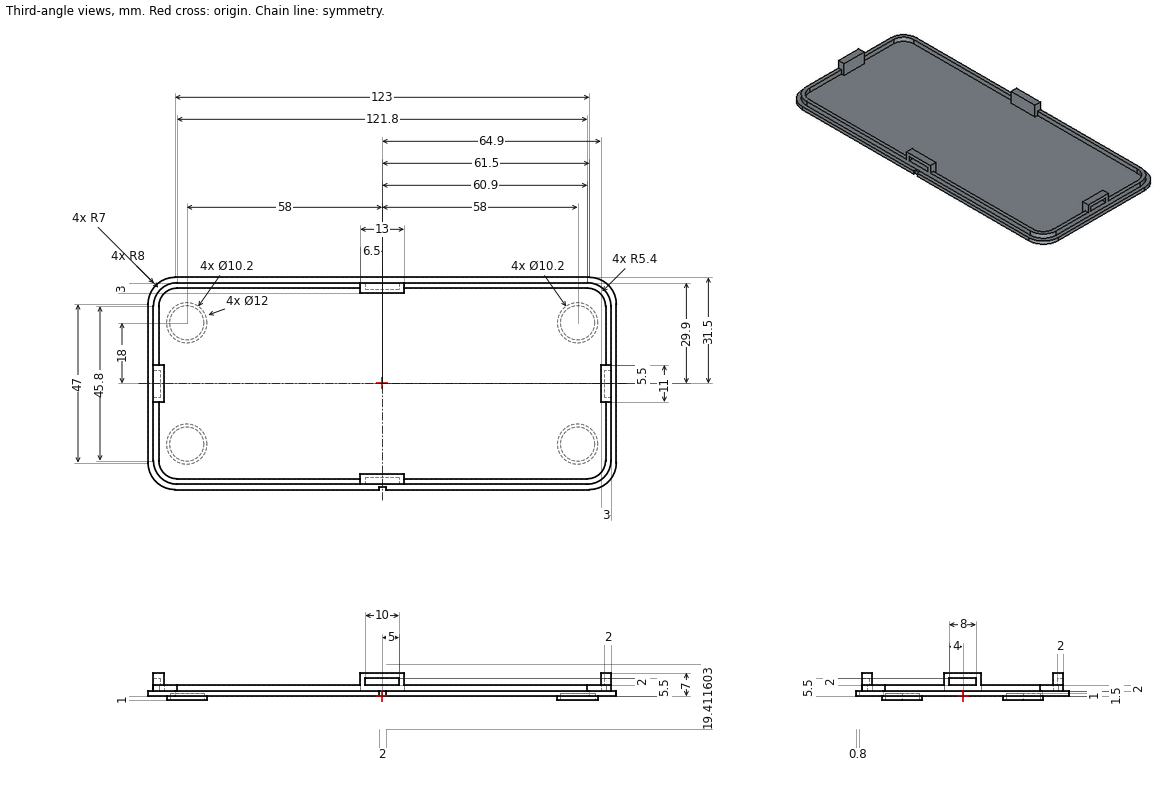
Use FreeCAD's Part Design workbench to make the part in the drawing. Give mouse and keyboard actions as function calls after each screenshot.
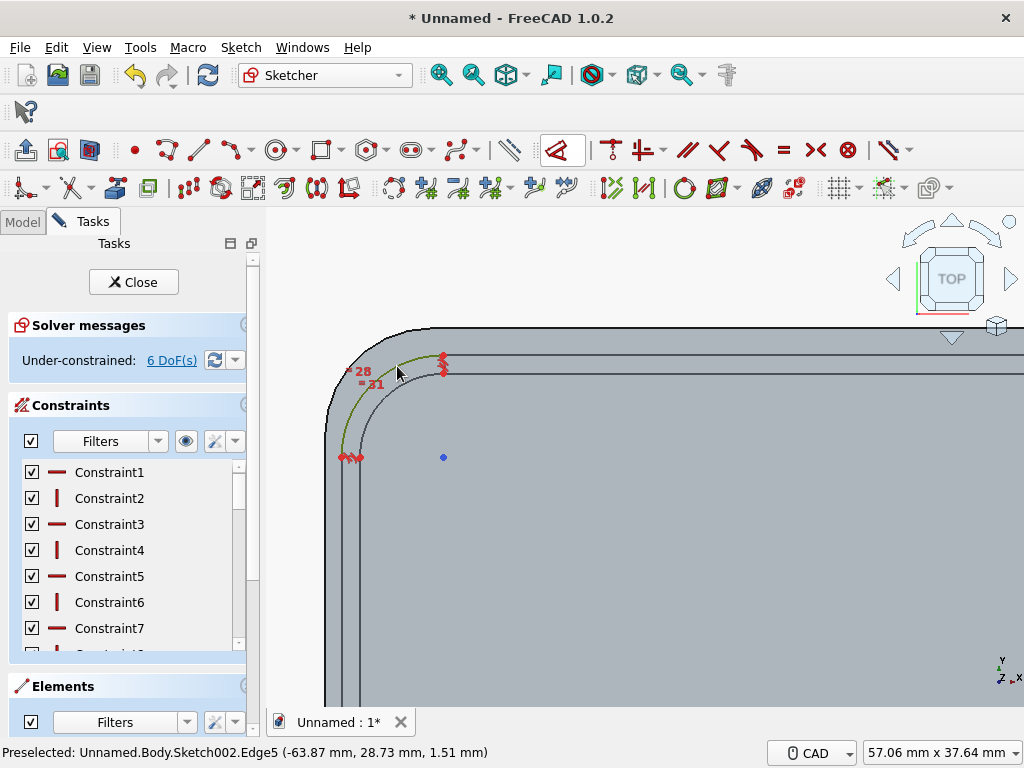
key(k)
key(r)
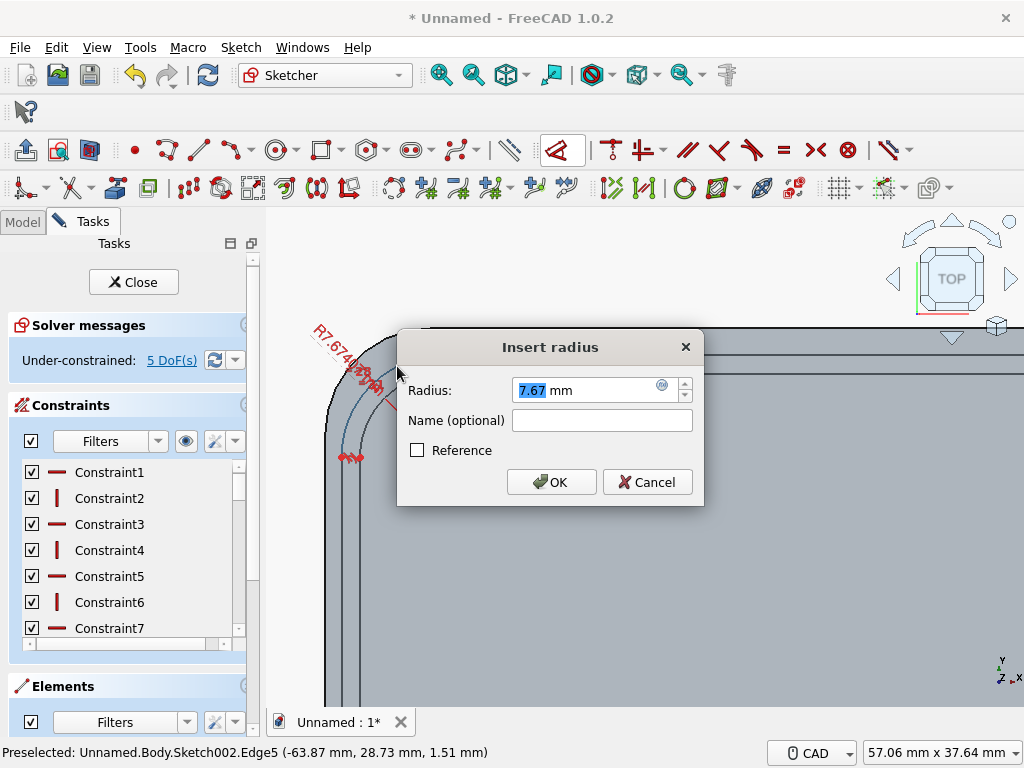
text(7)
key(Return)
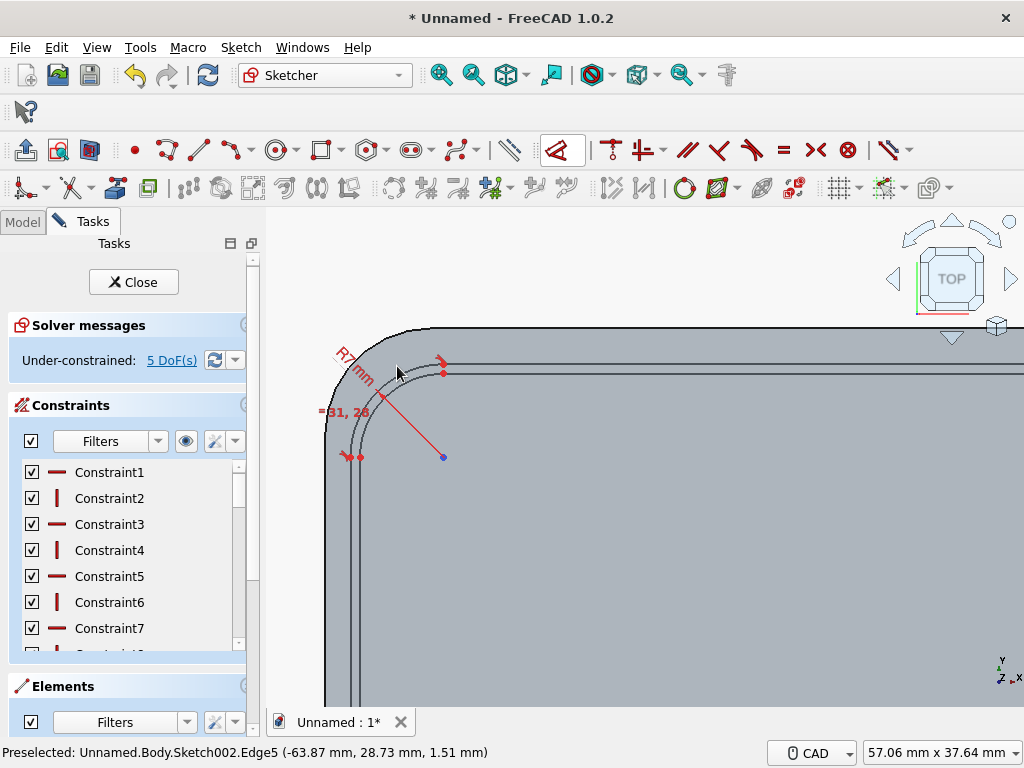
scroll(406, 384, down, 8)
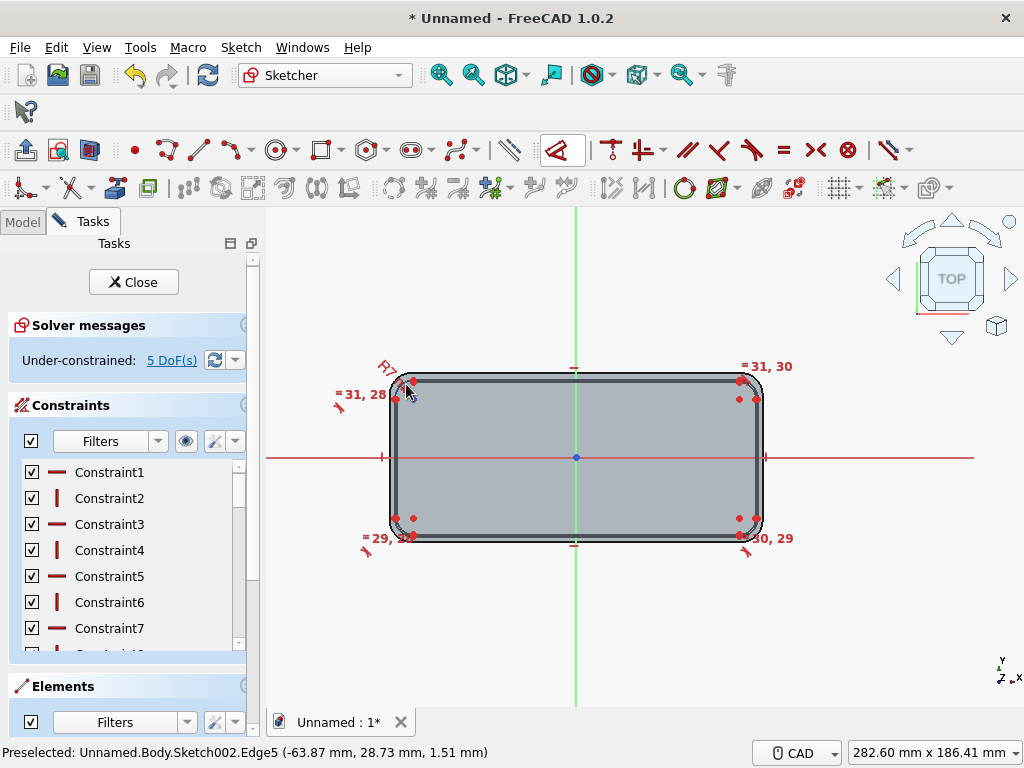
scroll(754, 391, up, 10)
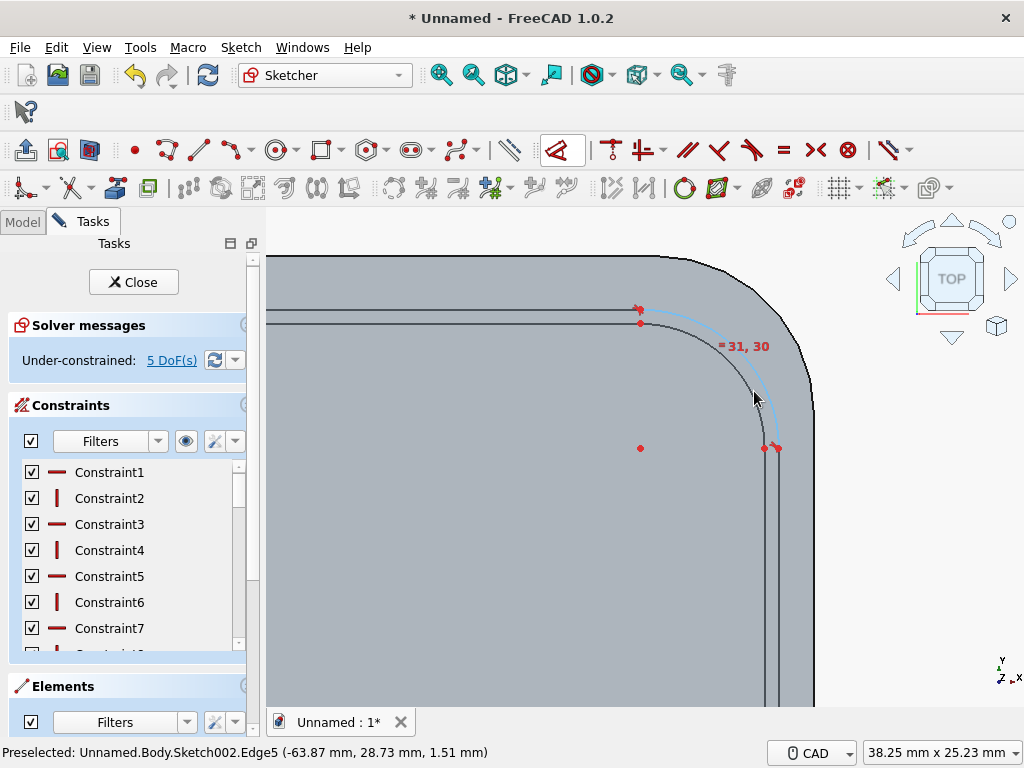
click(751, 392)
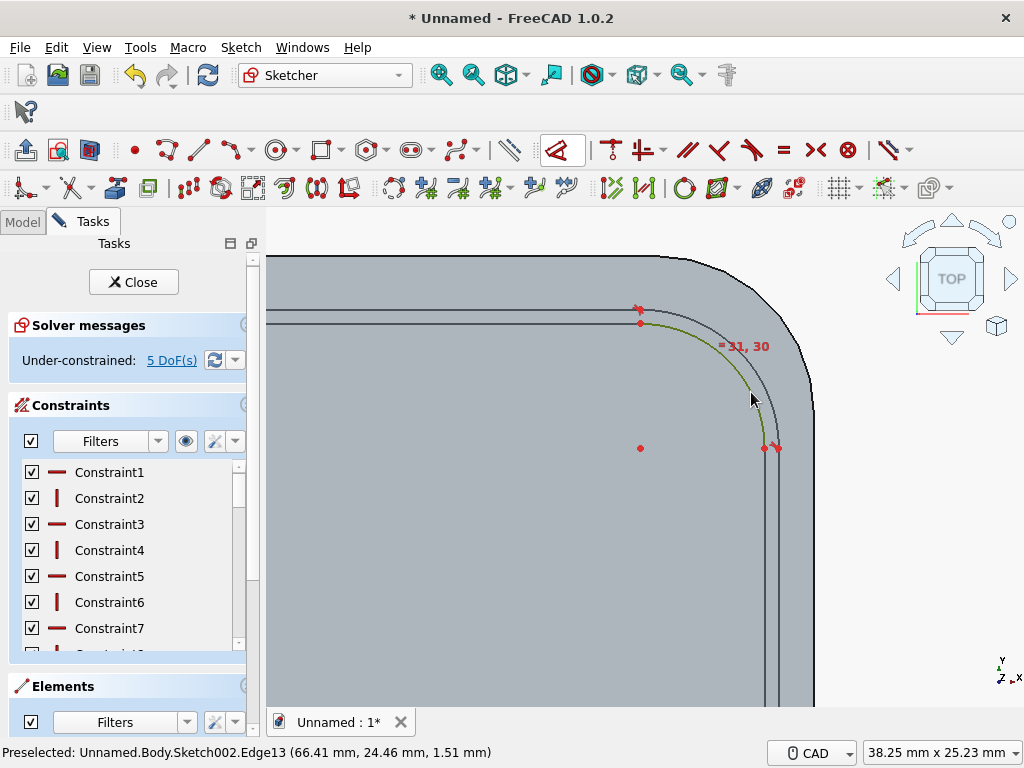
key(k)
key(r)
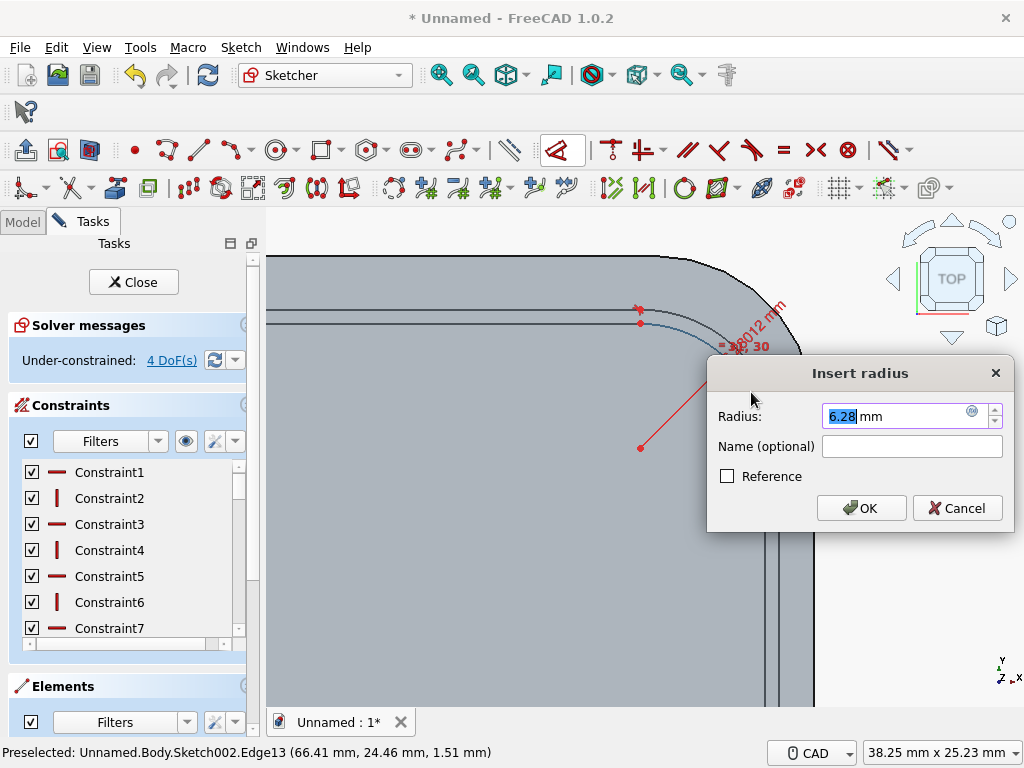
text(5.4)
key(Return)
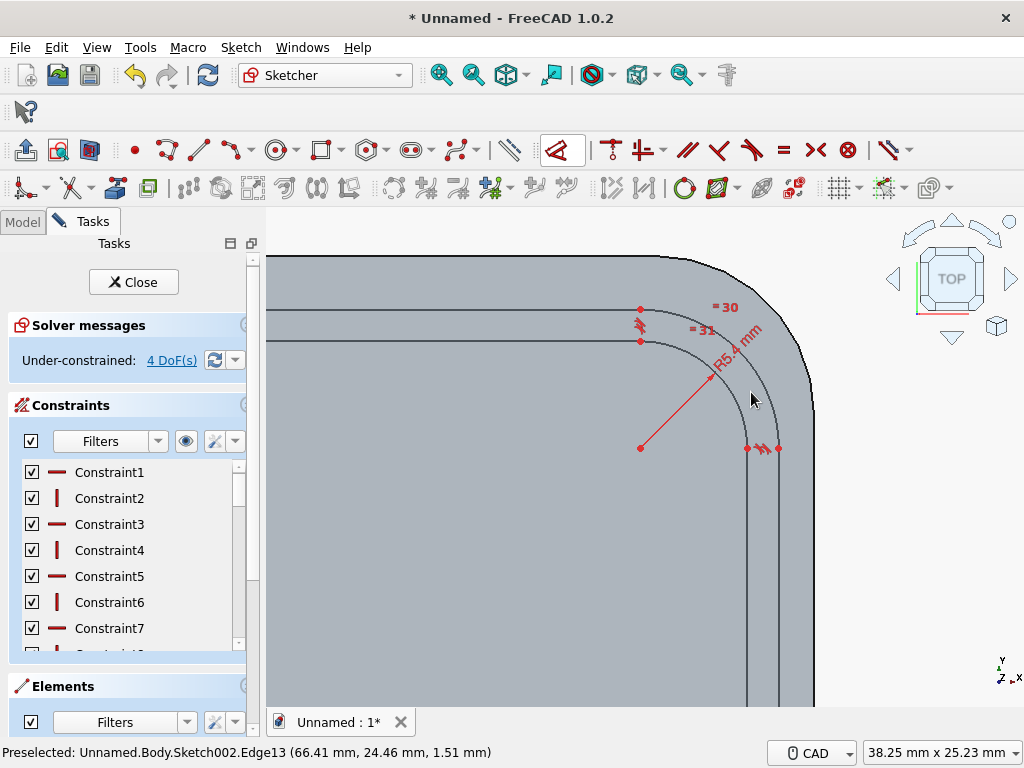
scroll(755, 391, down, 10)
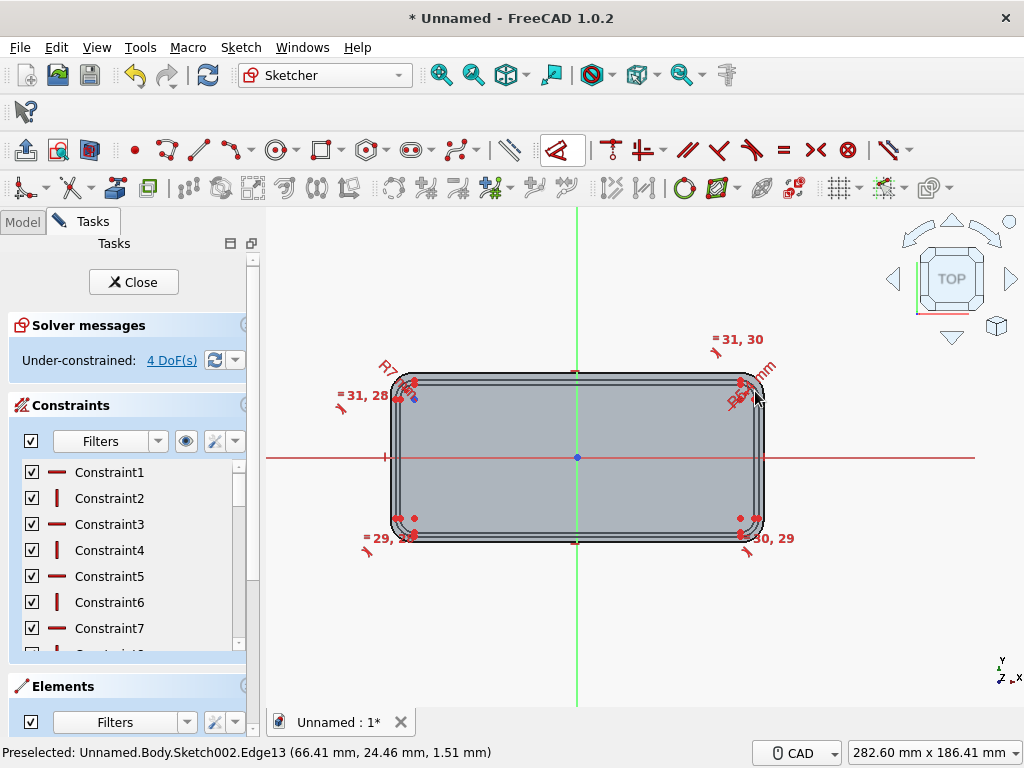
scroll(396, 435, up, 6)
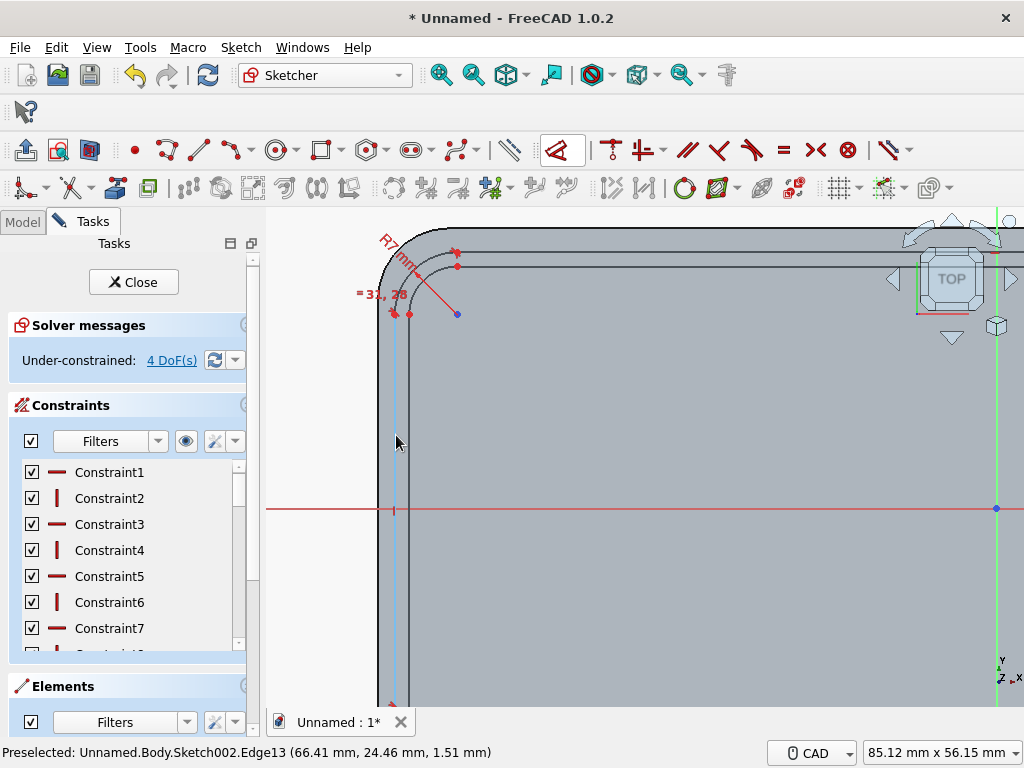
click(395, 433)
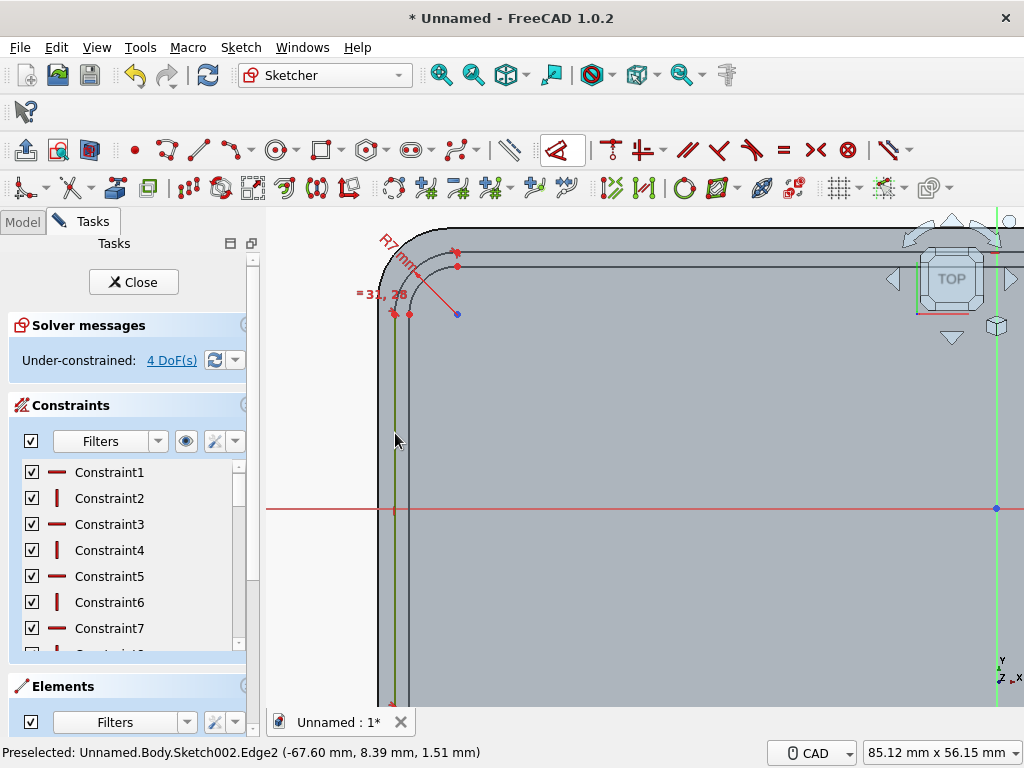
key(i)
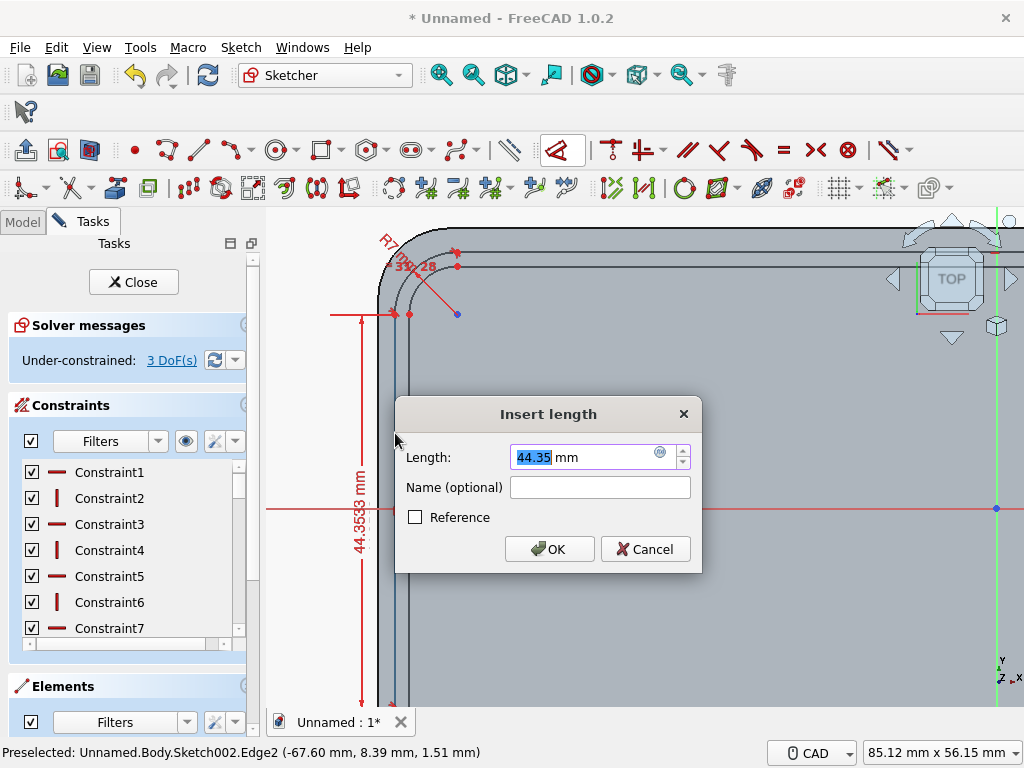
text(45.8)
key(Return)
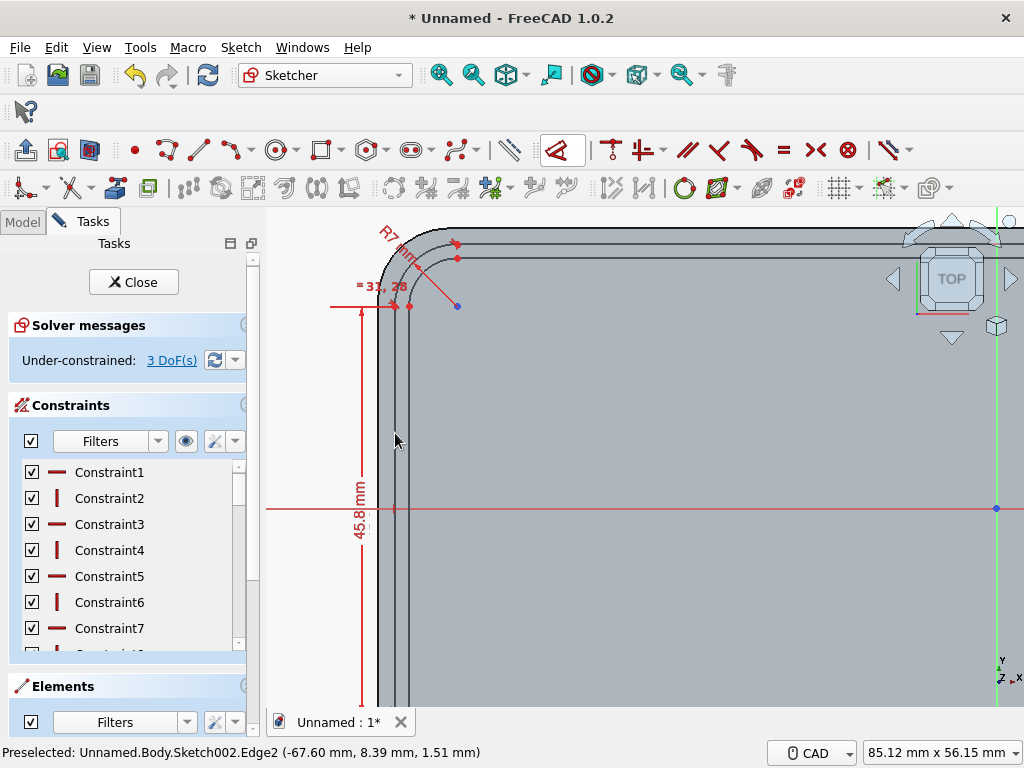
click(781, 244)